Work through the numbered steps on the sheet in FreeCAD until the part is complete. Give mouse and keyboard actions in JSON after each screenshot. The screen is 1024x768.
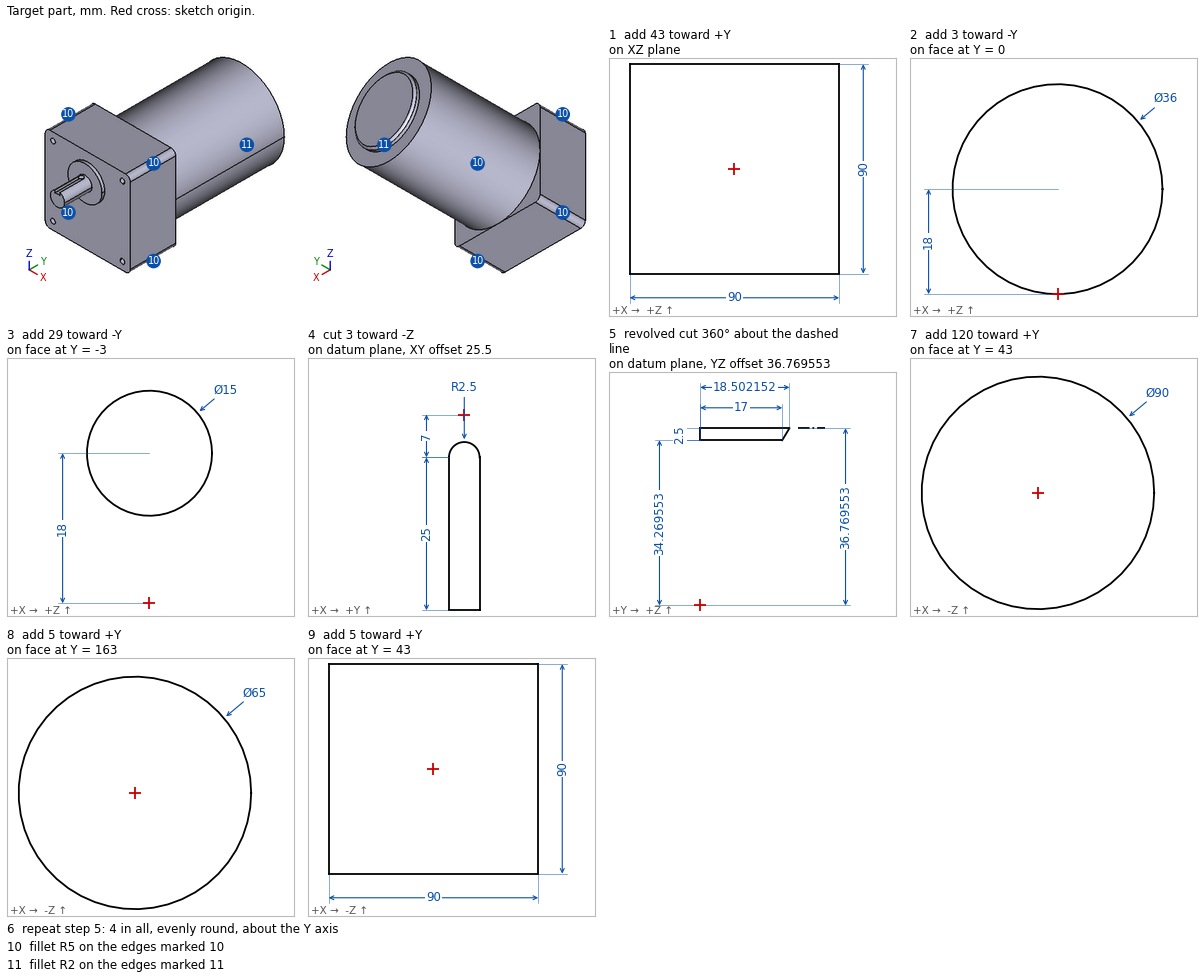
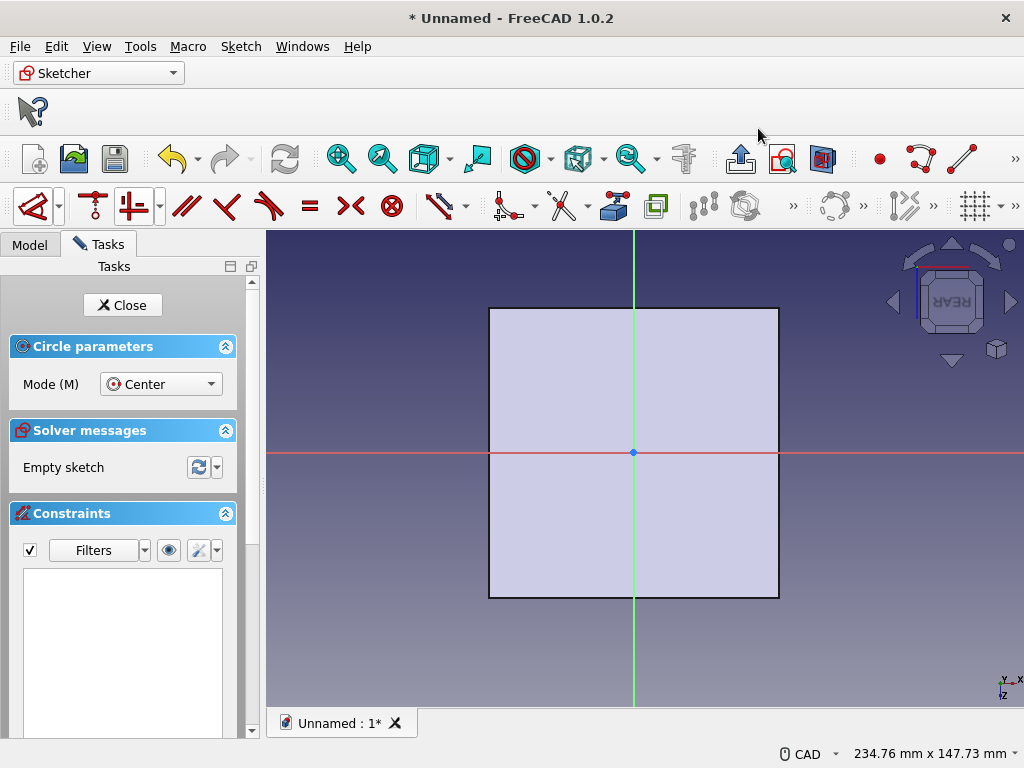
{"action": "left_click", "coordinate": [634, 453]}
{"action": "mouse_move", "coordinate": [737, 350]}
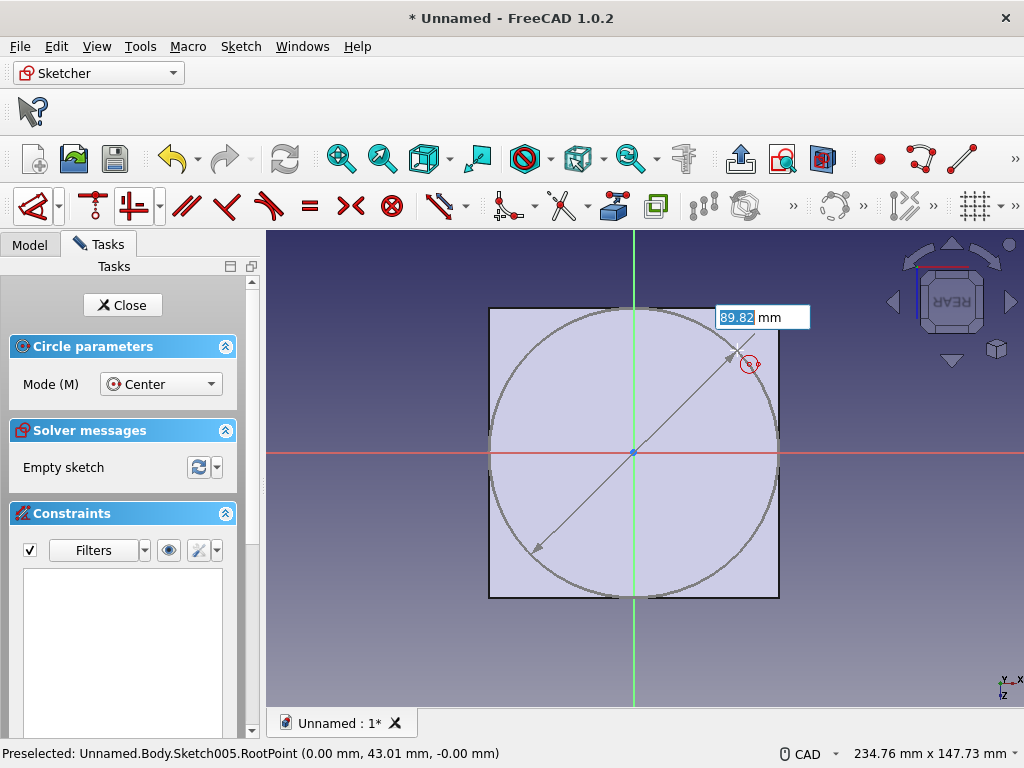
{"action": "type", "text": "90"}
{"action": "key", "text": "Return"}
{"action": "key", "text": "Escape"}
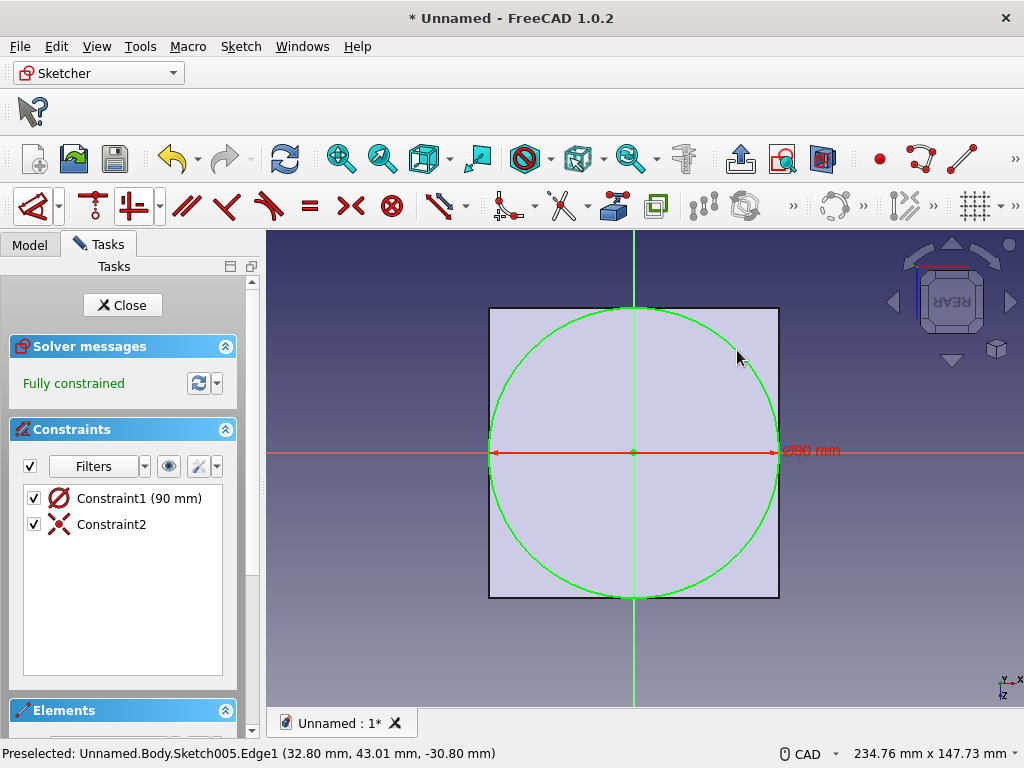
{"action": "left_click", "coordinate": [123, 305]}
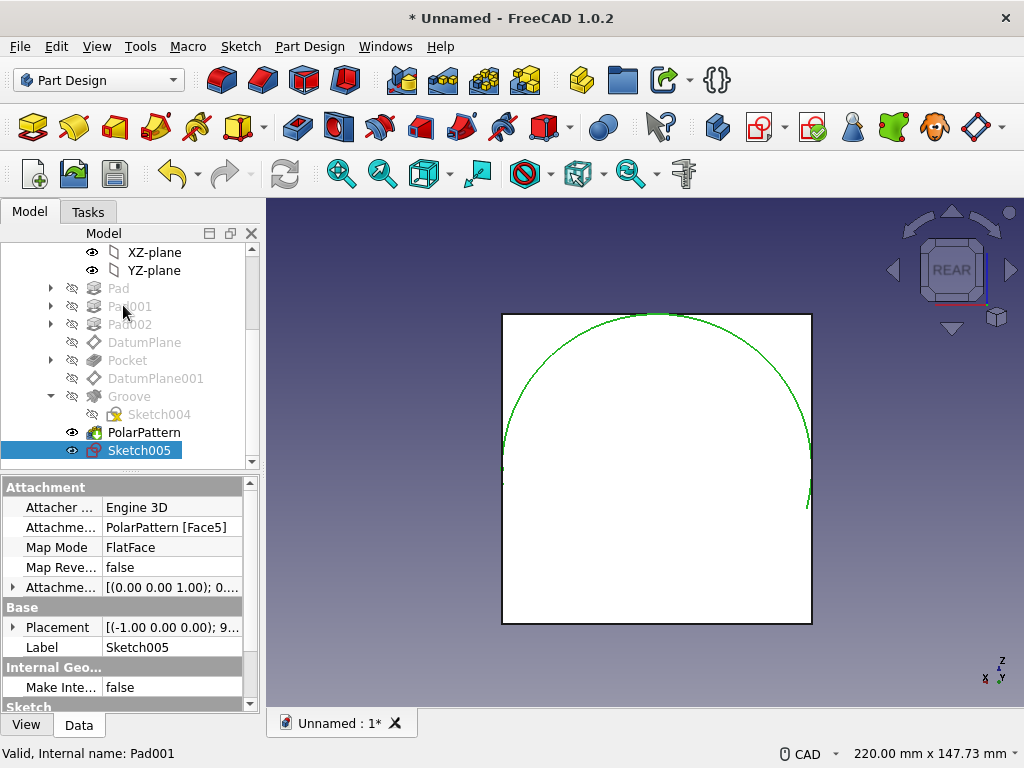
{"action": "left_click", "coordinate": [33, 128]}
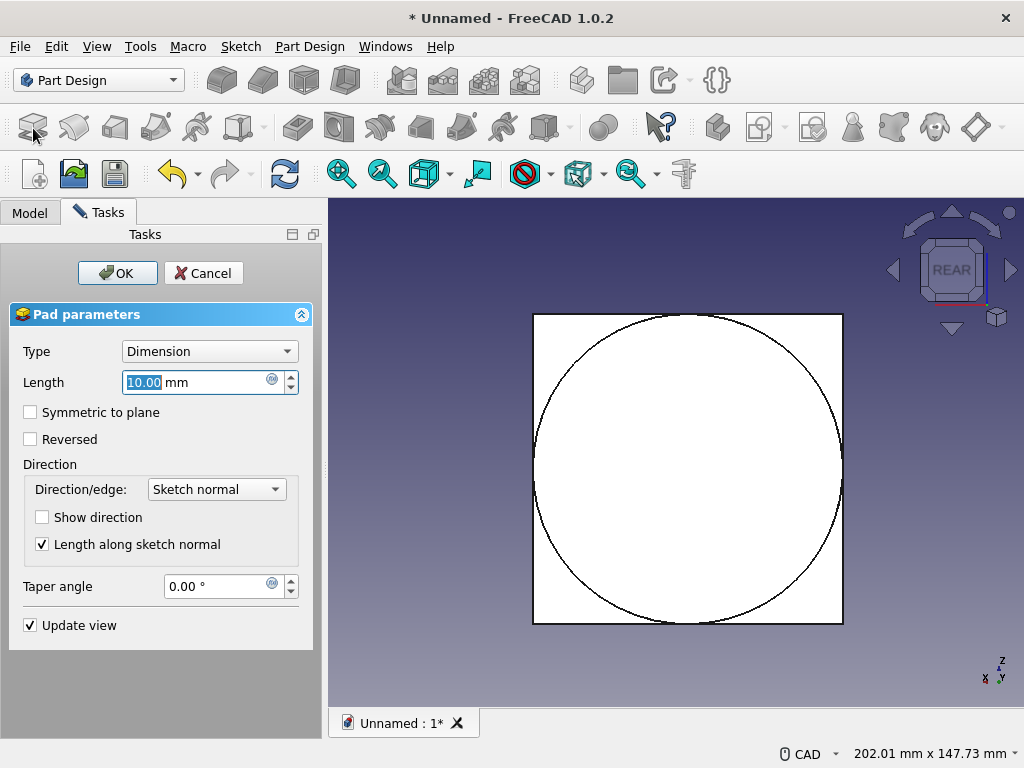
{"action": "type", "text": "120"}
{"action": "key", "text": "Tab"}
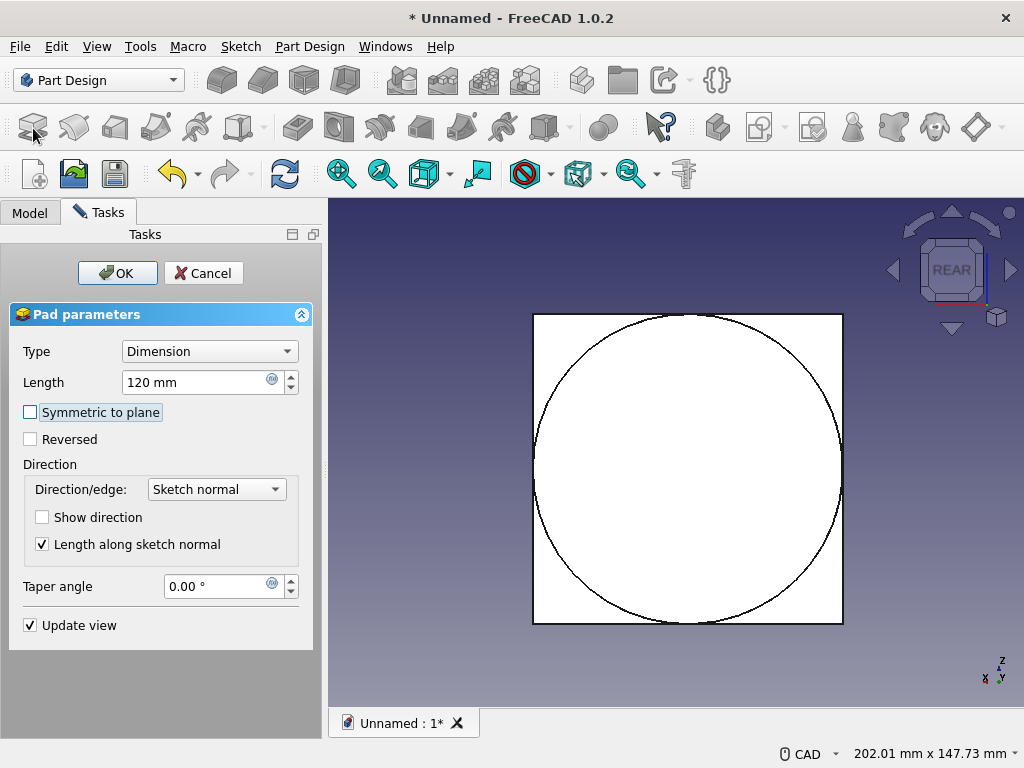
{"action": "left_click", "coordinate": [118, 273]}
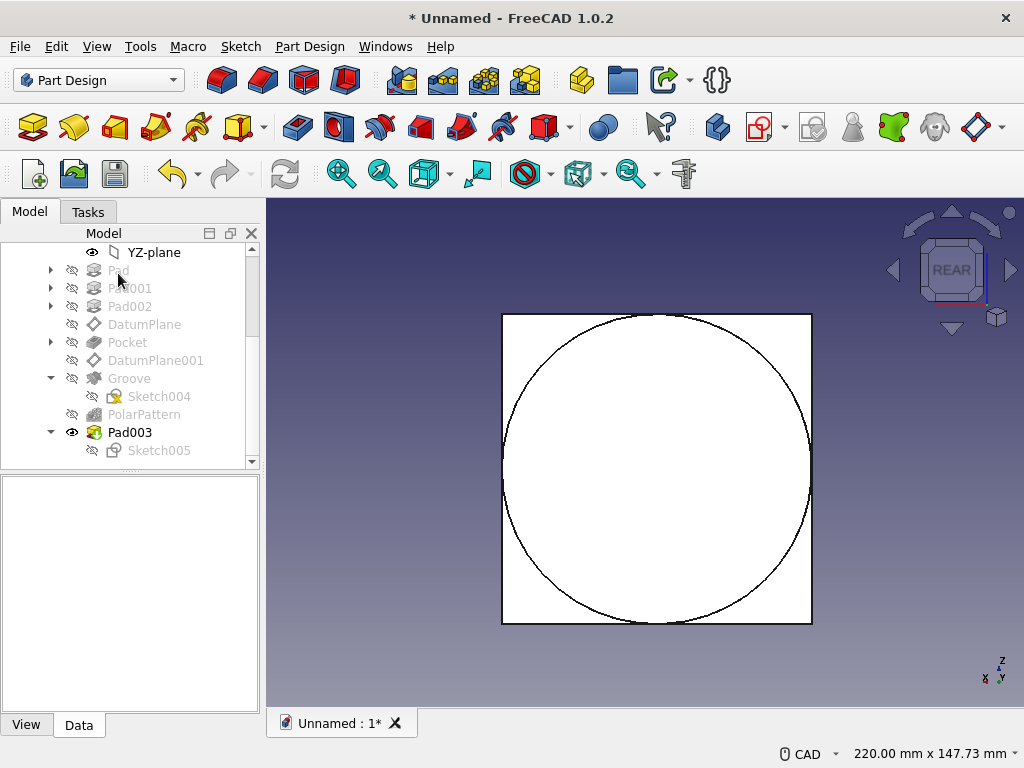
{"action": "left_click", "coordinate": [657, 468]}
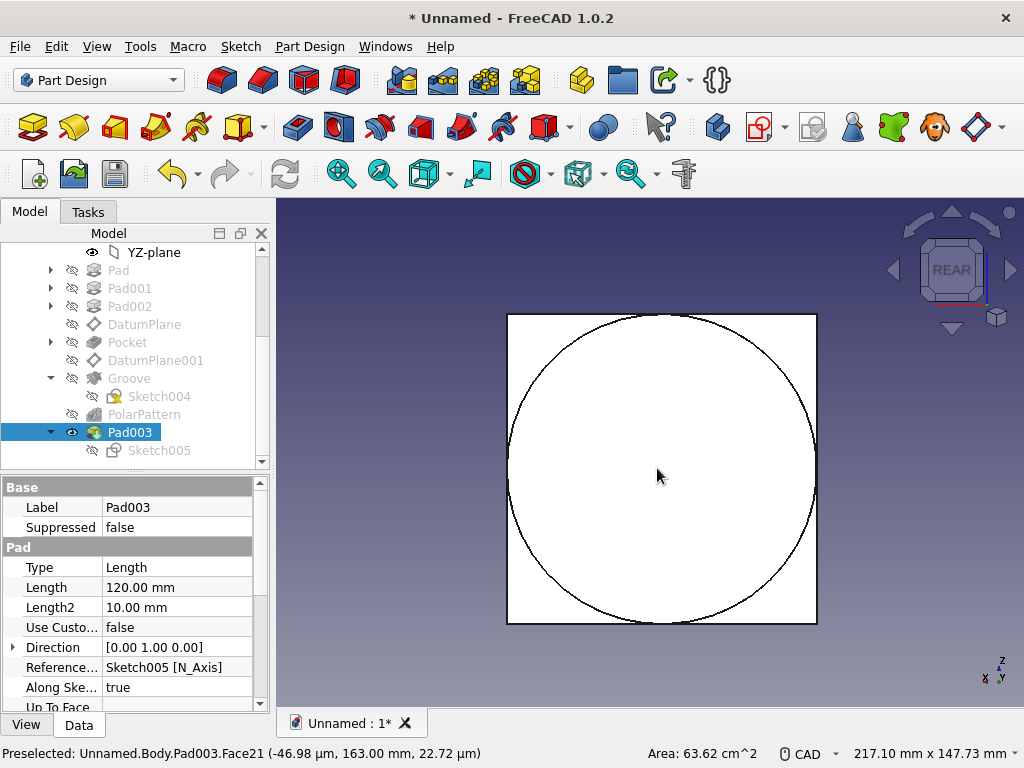
{"action": "left_click", "coordinate": [758, 128]}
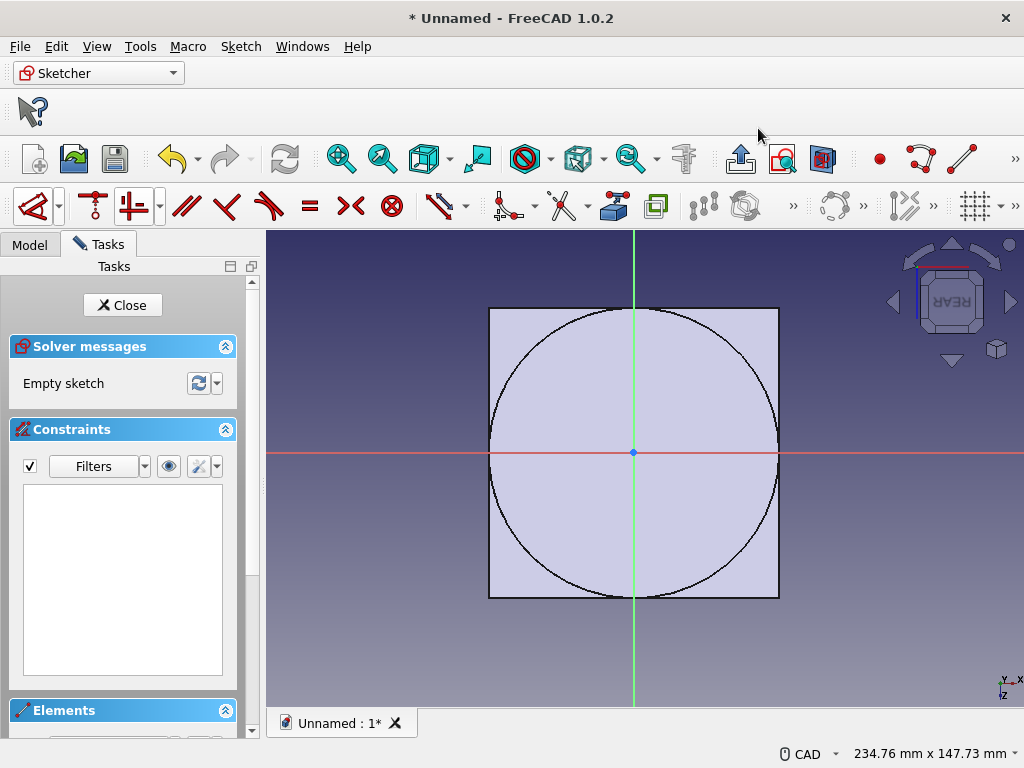
{"action": "scroll", "coordinate": [751, 421], "scroll_direction": "up", "scroll_amount": 2}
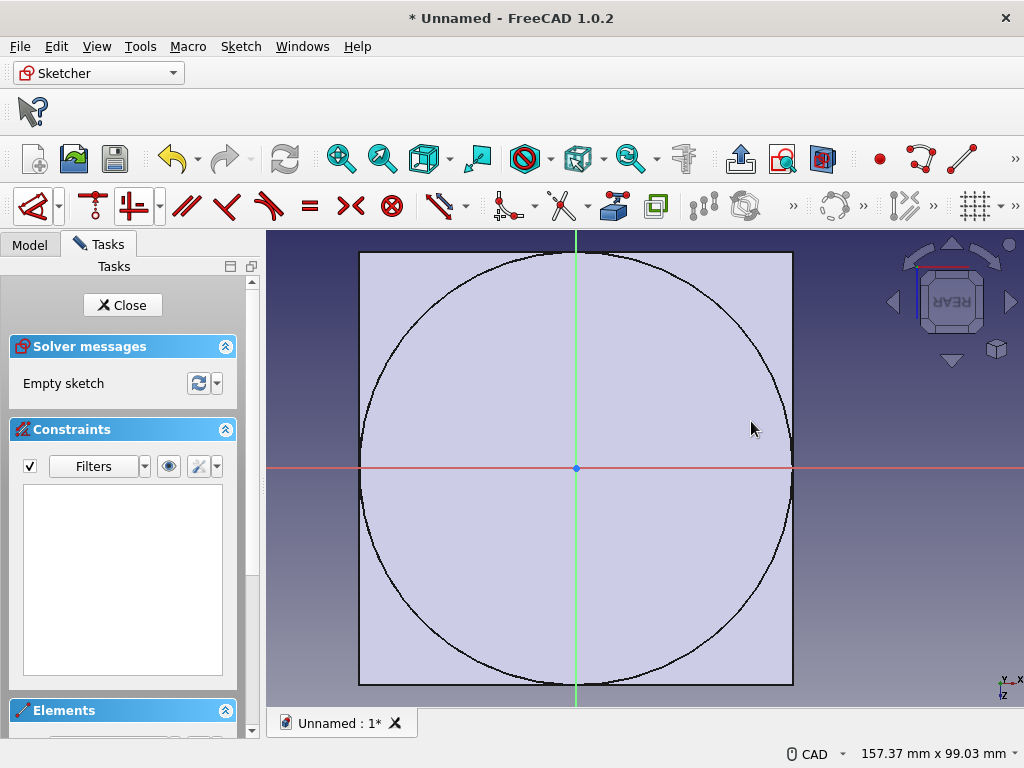
{"action": "key", "text": "g c"}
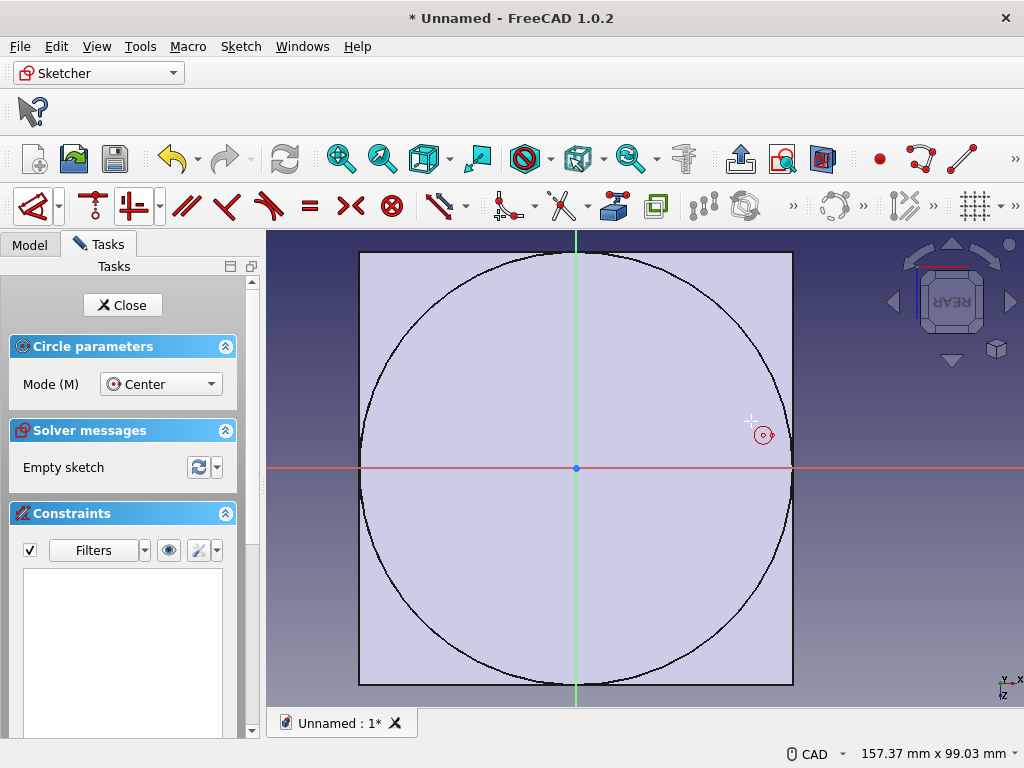
{"action": "left_click", "coordinate": [576, 468]}
{"action": "mouse_move", "coordinate": [687, 358]}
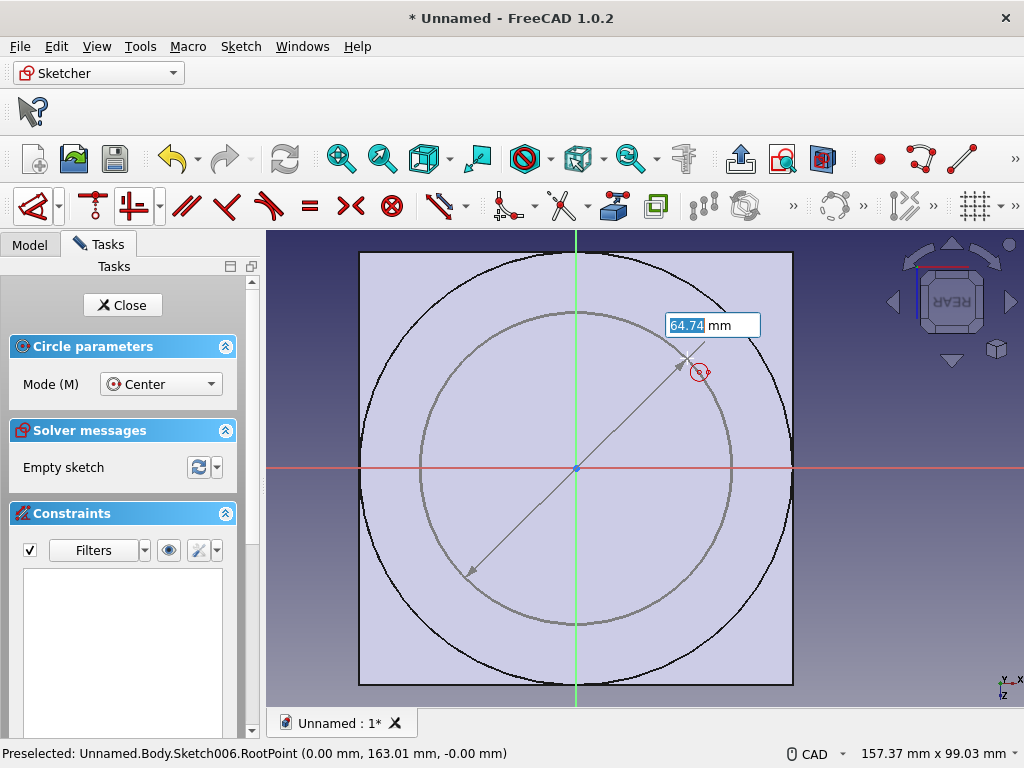
{"action": "type", "text": "65"}
{"action": "key", "text": "Return"}
{"action": "key", "text": "Escape"}